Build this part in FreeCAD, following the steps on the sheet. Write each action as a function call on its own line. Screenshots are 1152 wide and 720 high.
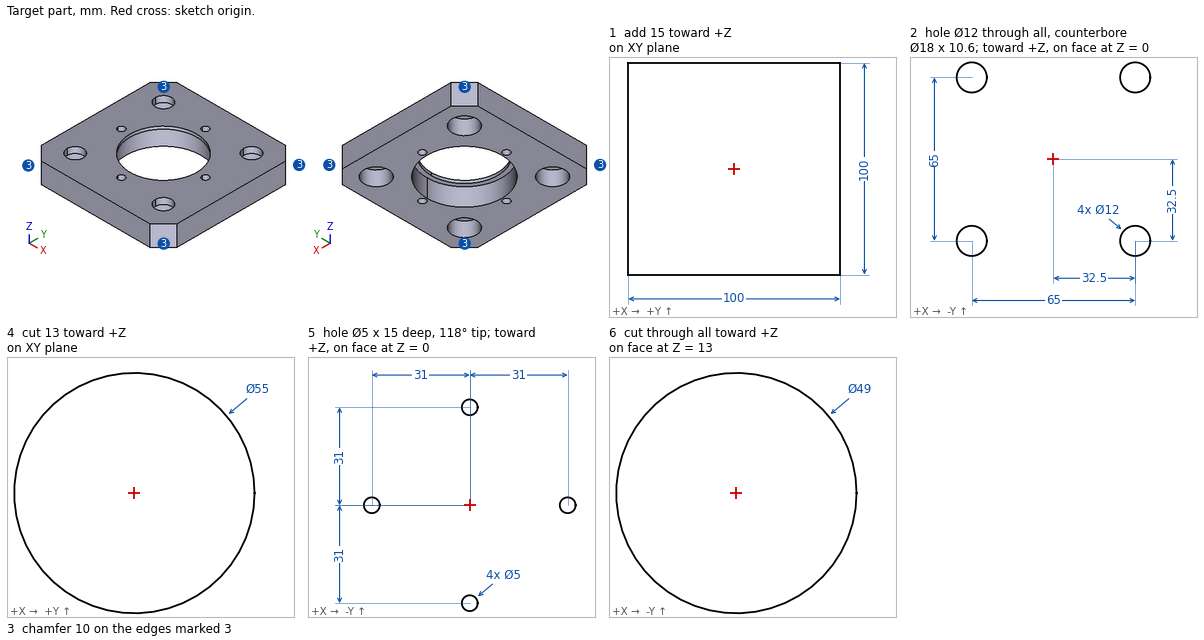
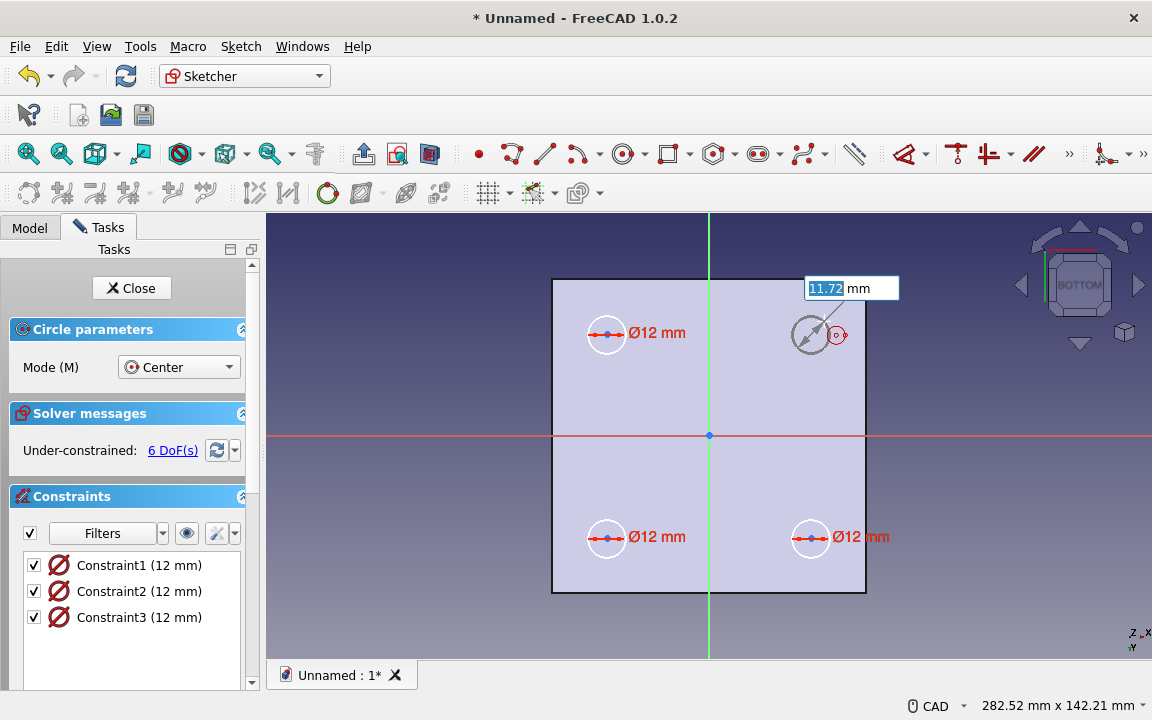
text(12)
key(Return)
key(Escape)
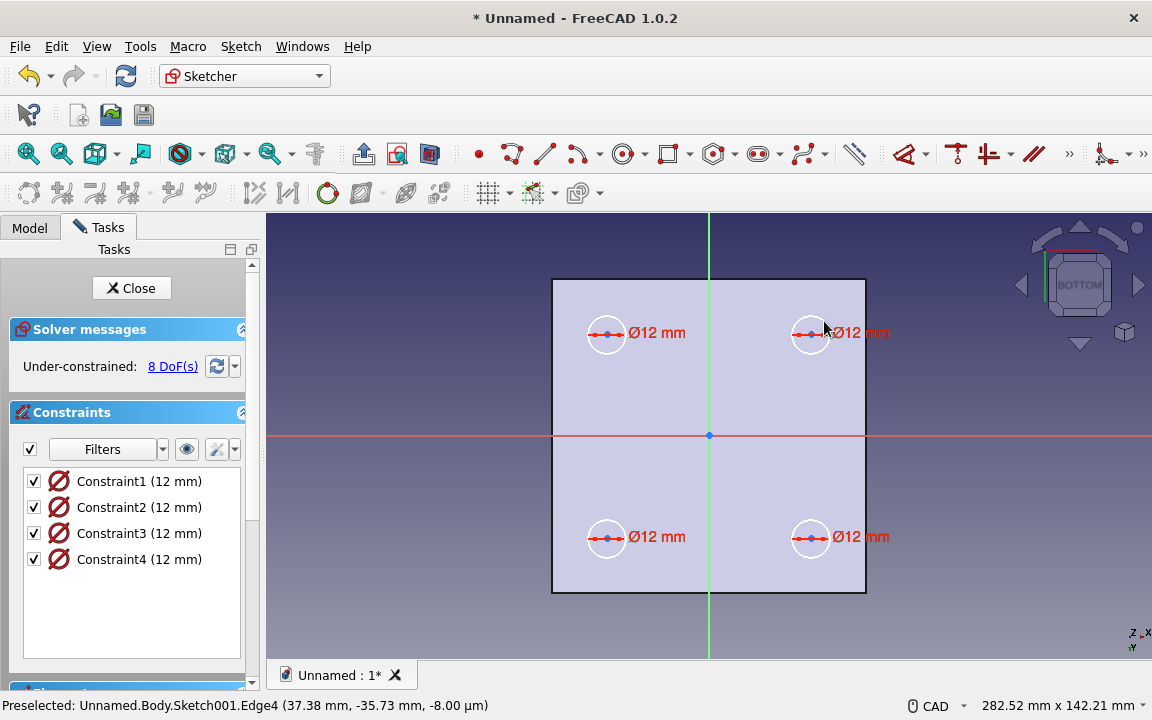
click(811, 539)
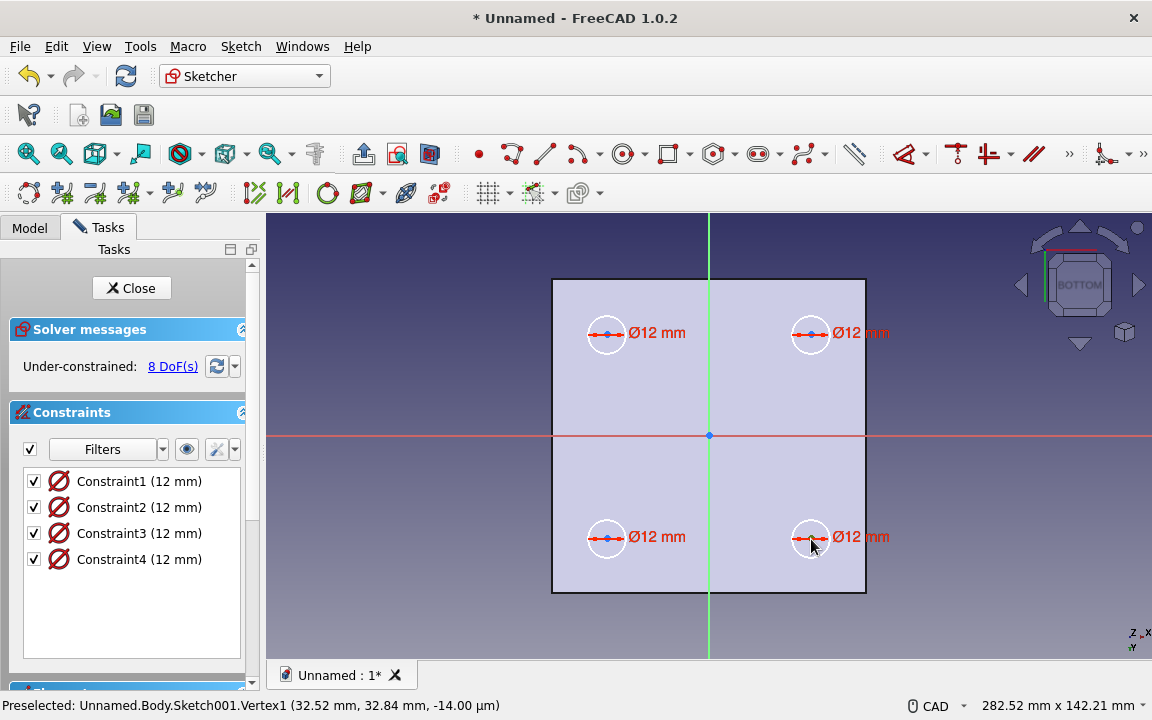
click(607, 539)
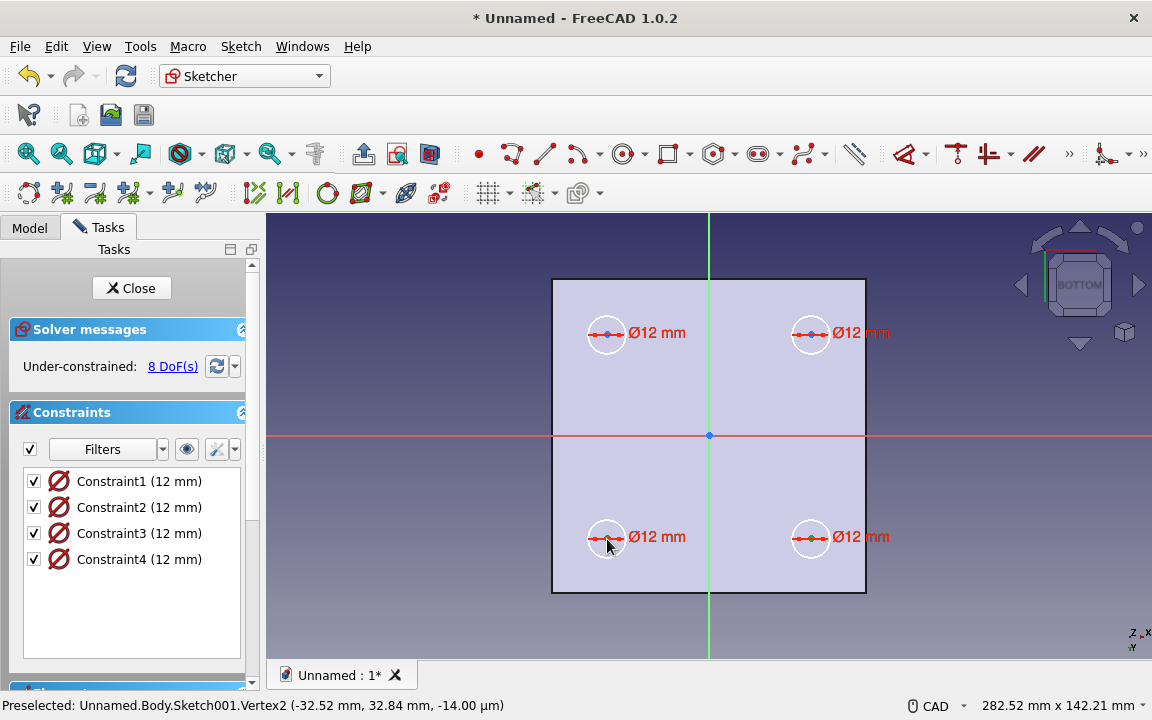
key(h)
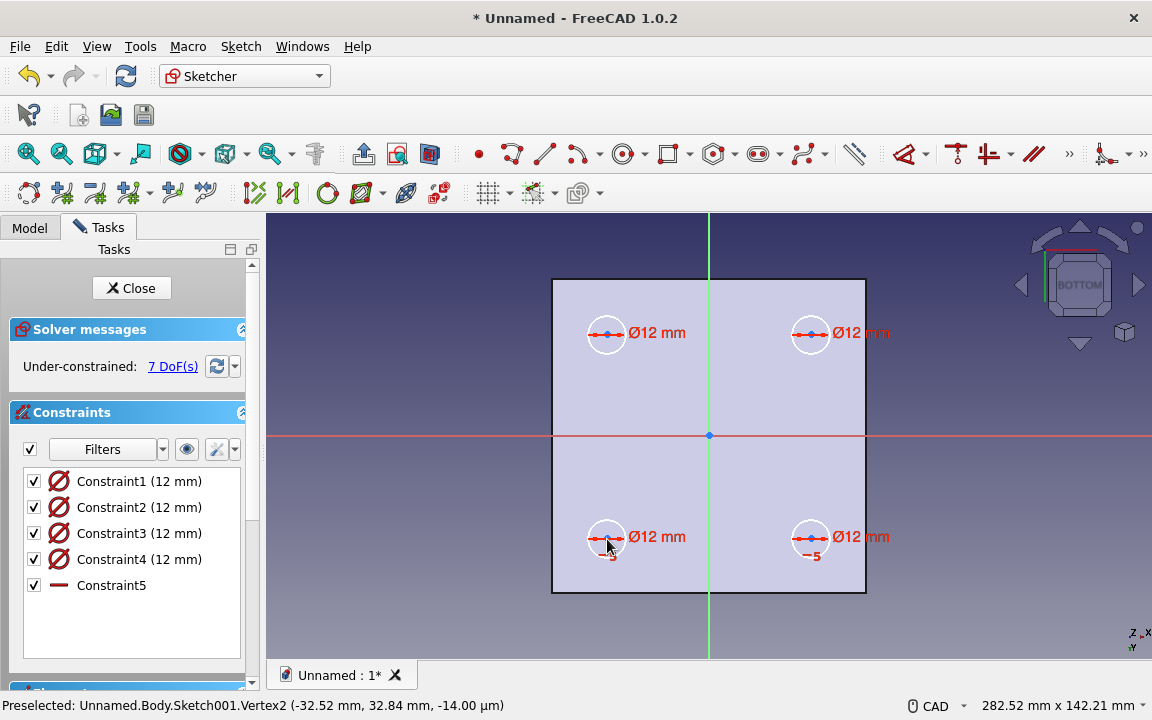
click(607, 539)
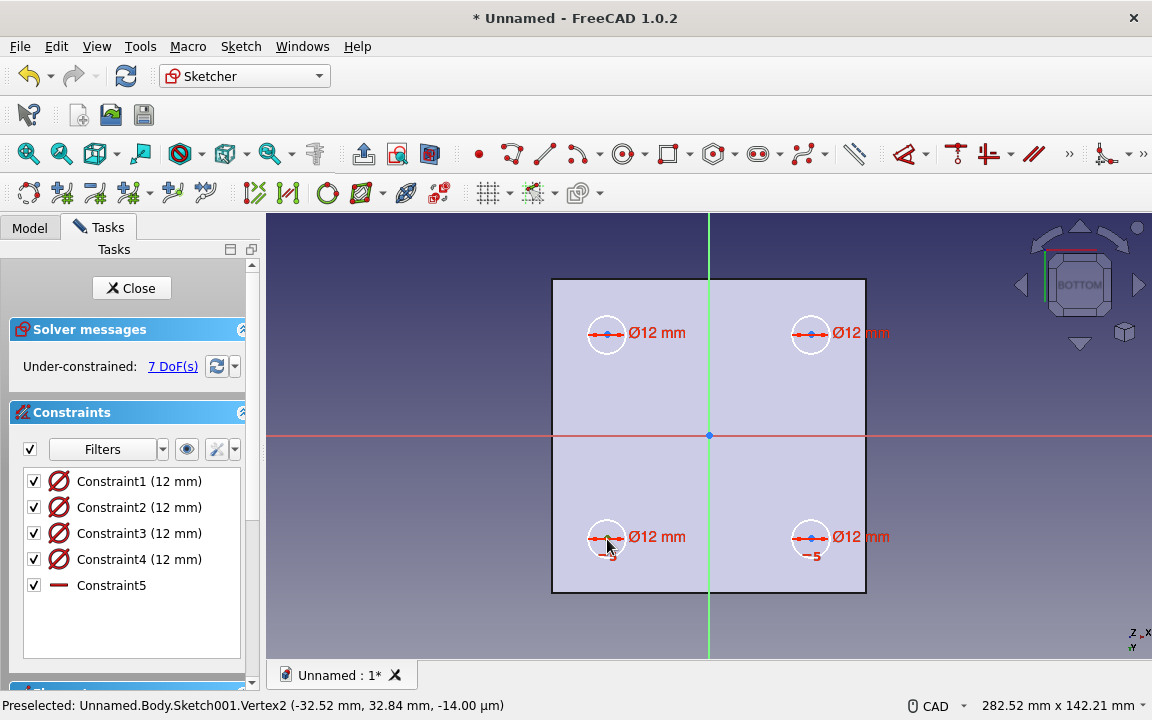
click(607, 335)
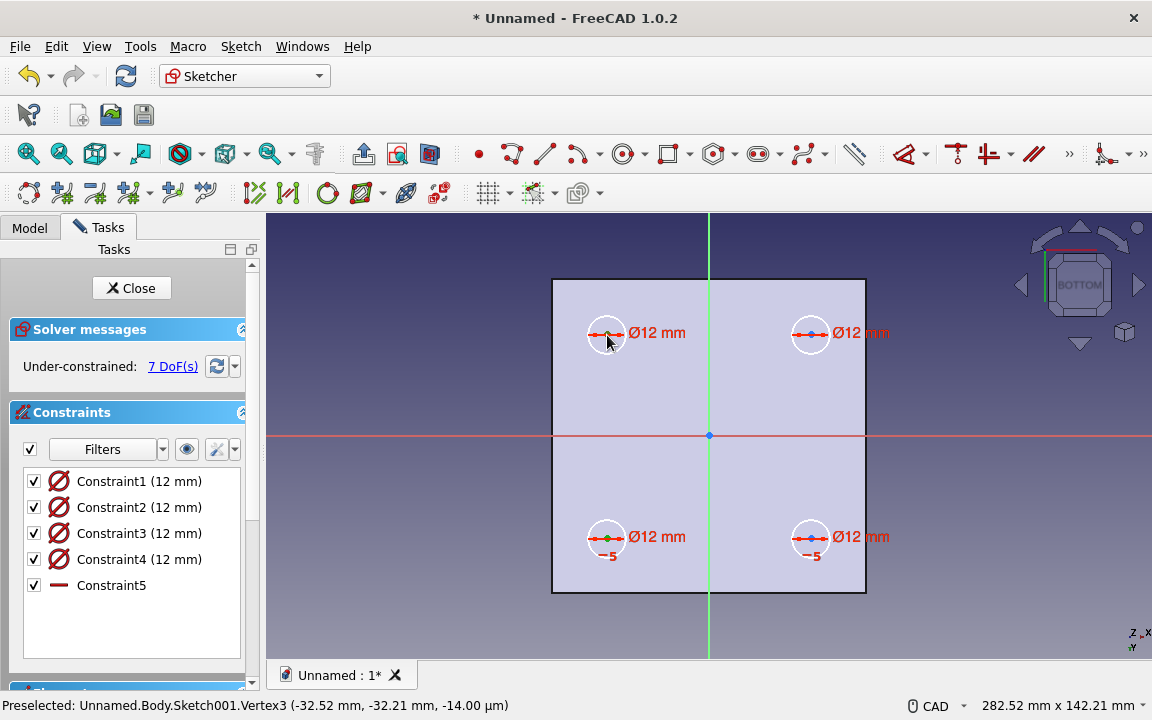
key(v)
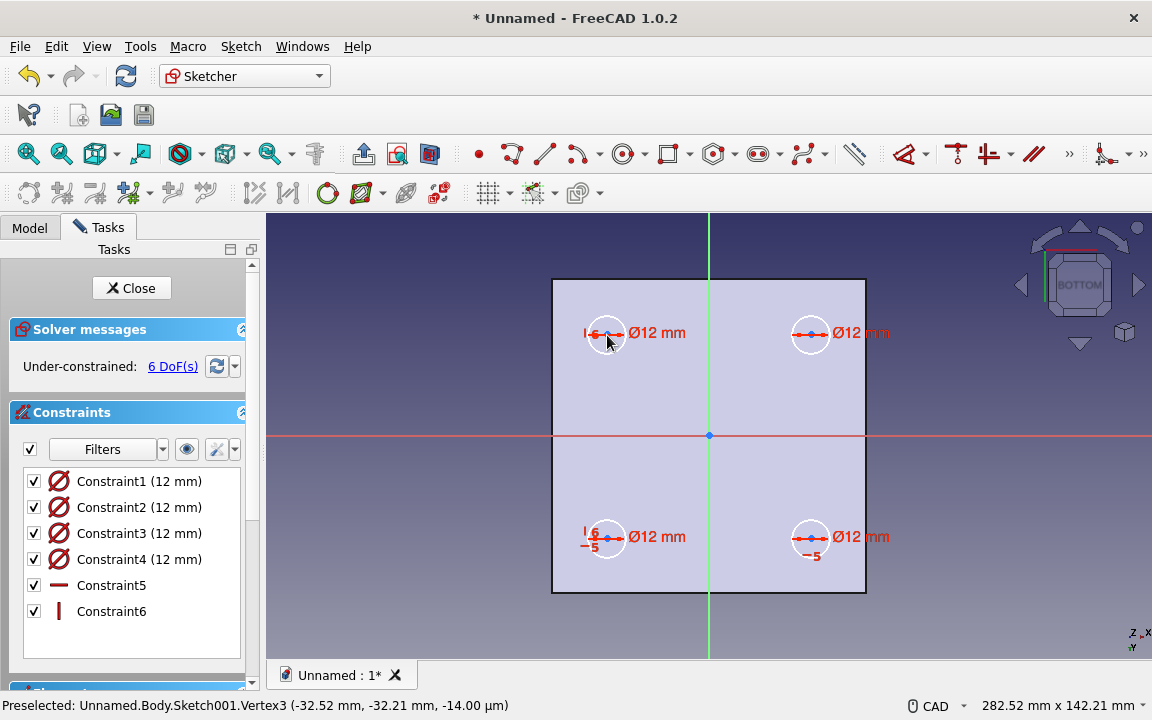
click(811, 539)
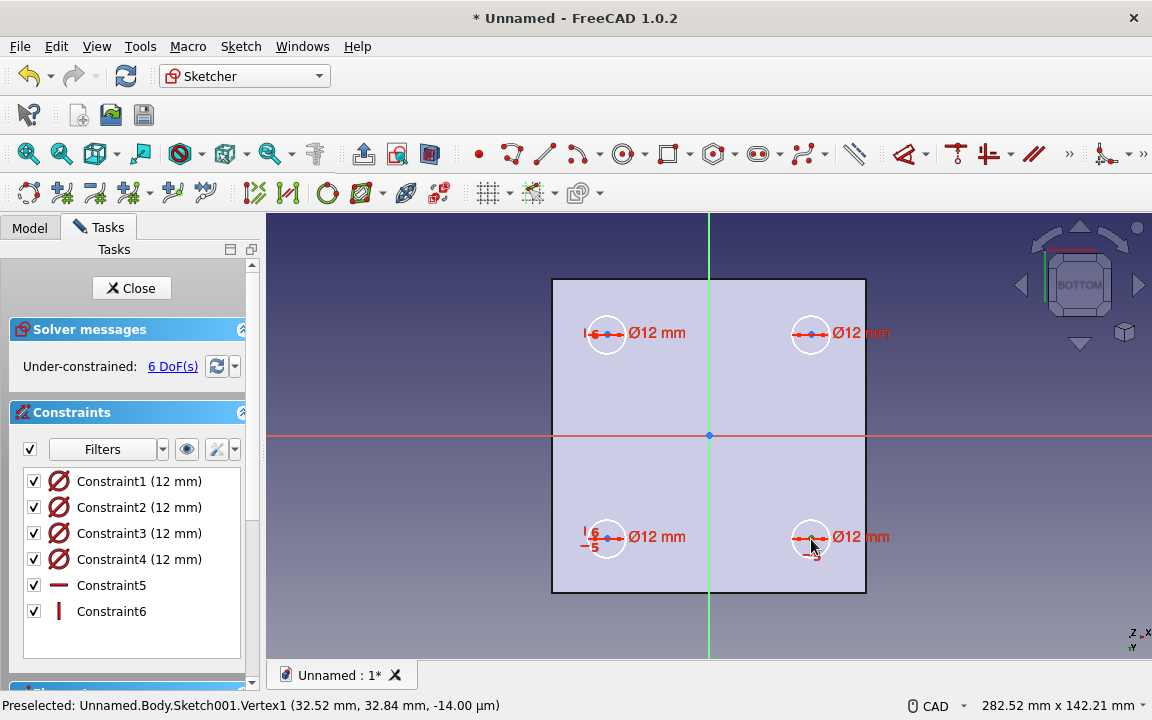
click(811, 335)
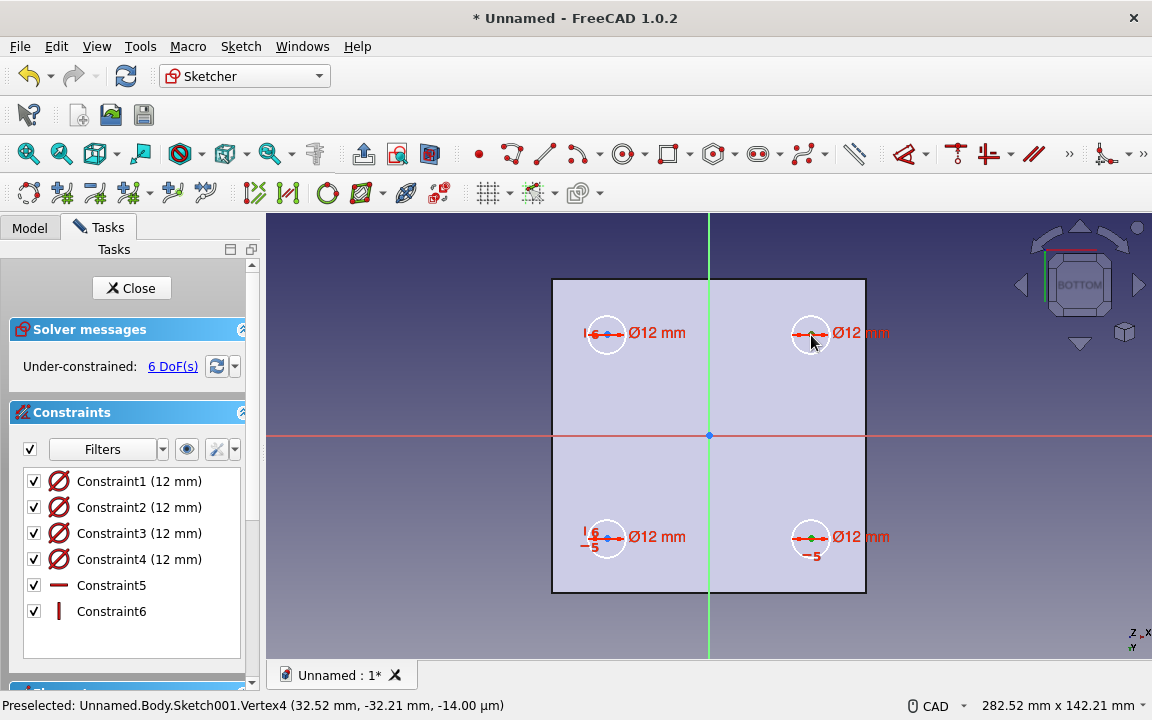
click(1010, 154)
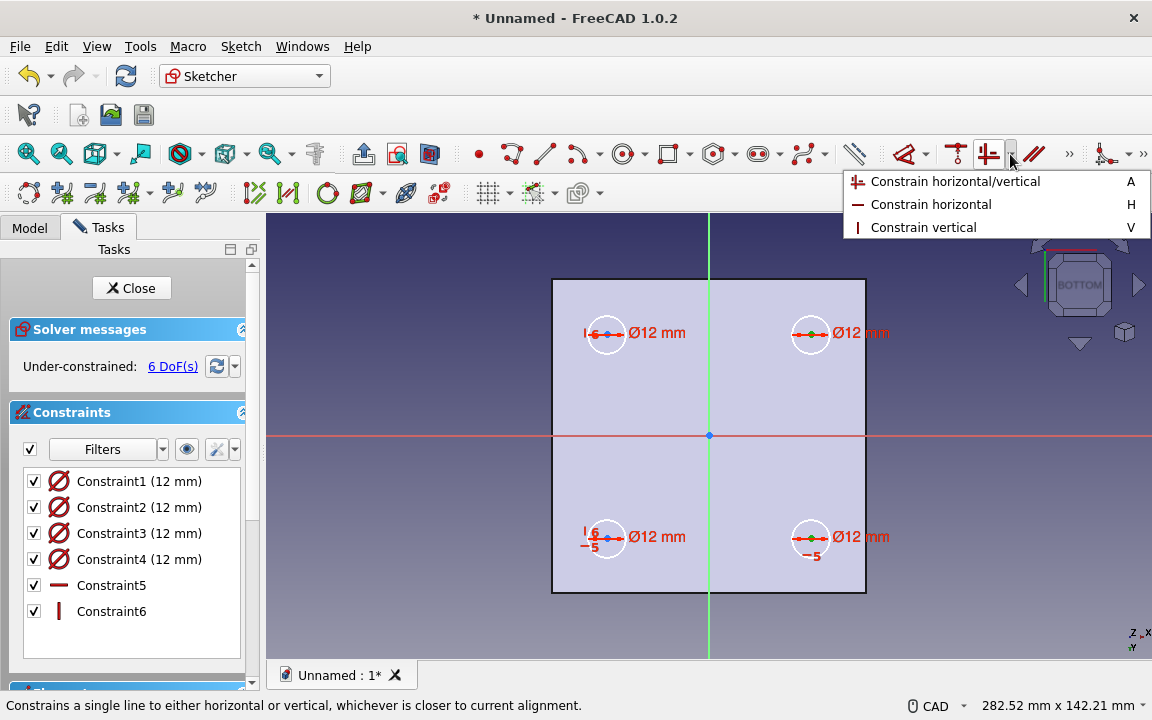
click(997, 228)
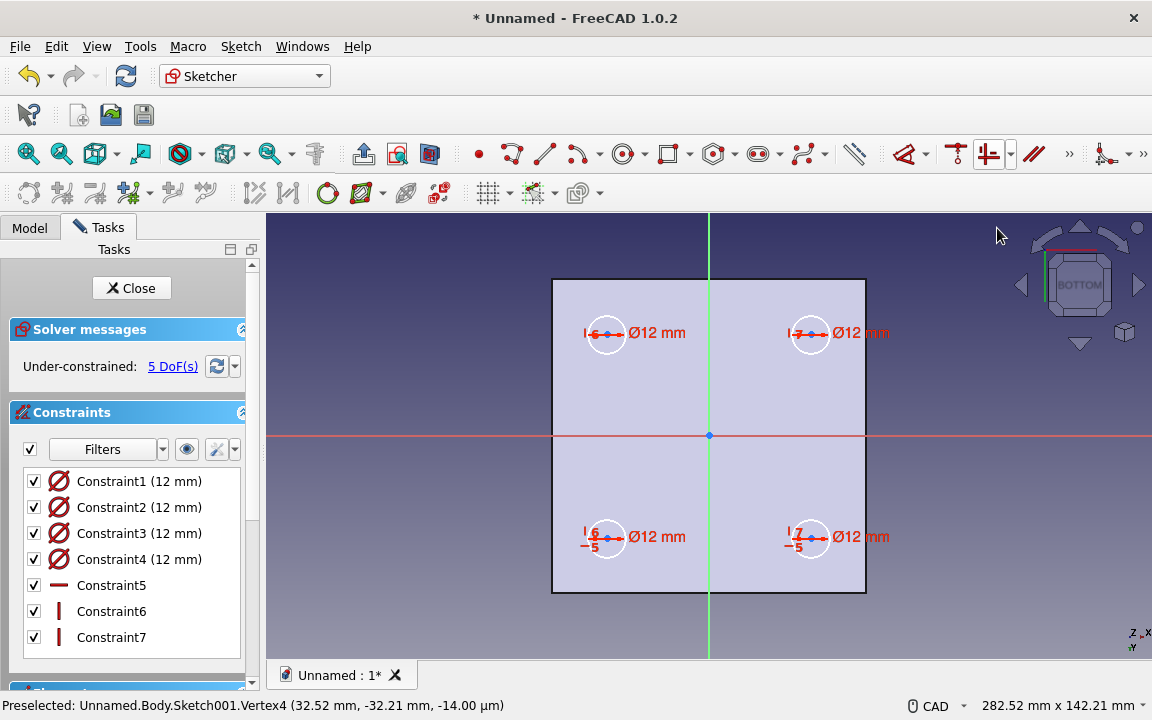
click(607, 335)